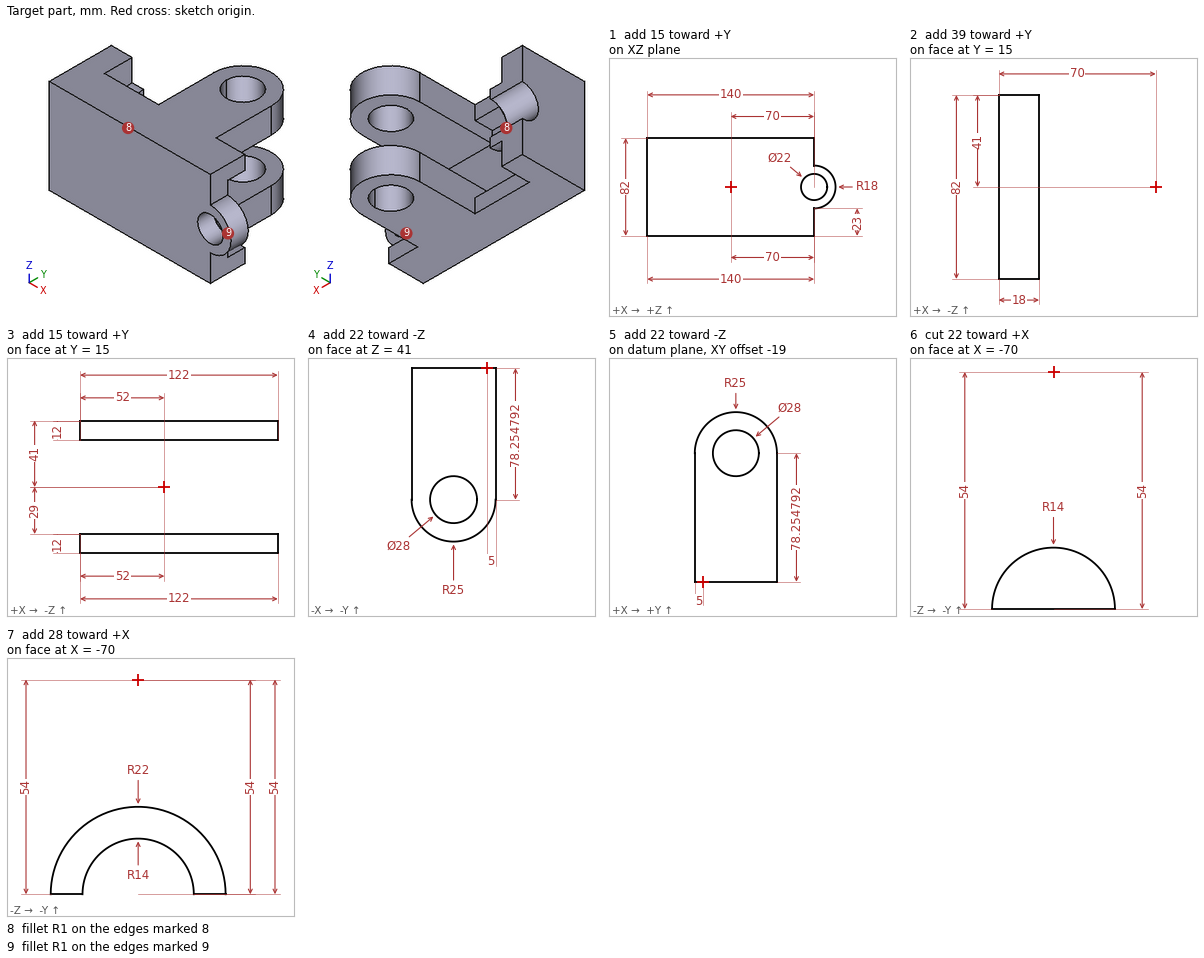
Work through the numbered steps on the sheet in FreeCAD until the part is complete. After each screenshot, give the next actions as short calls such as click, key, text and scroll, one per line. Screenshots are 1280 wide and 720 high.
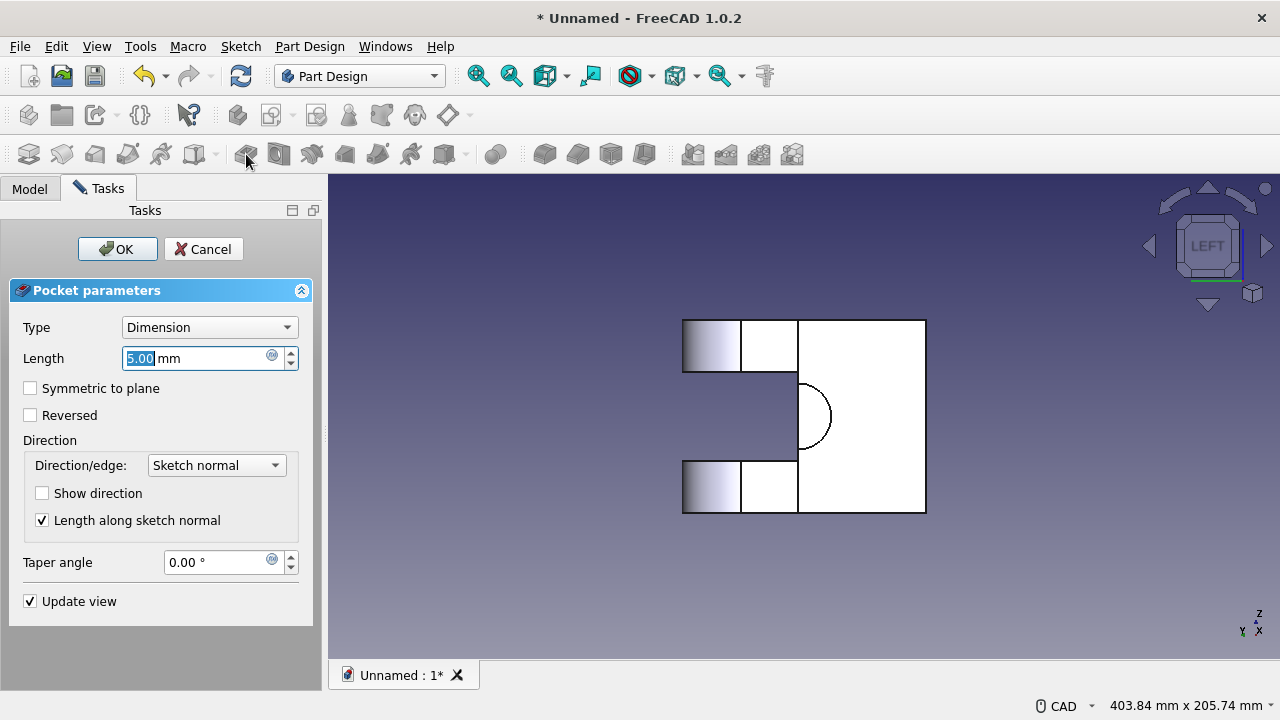
text(22)
key(Tab)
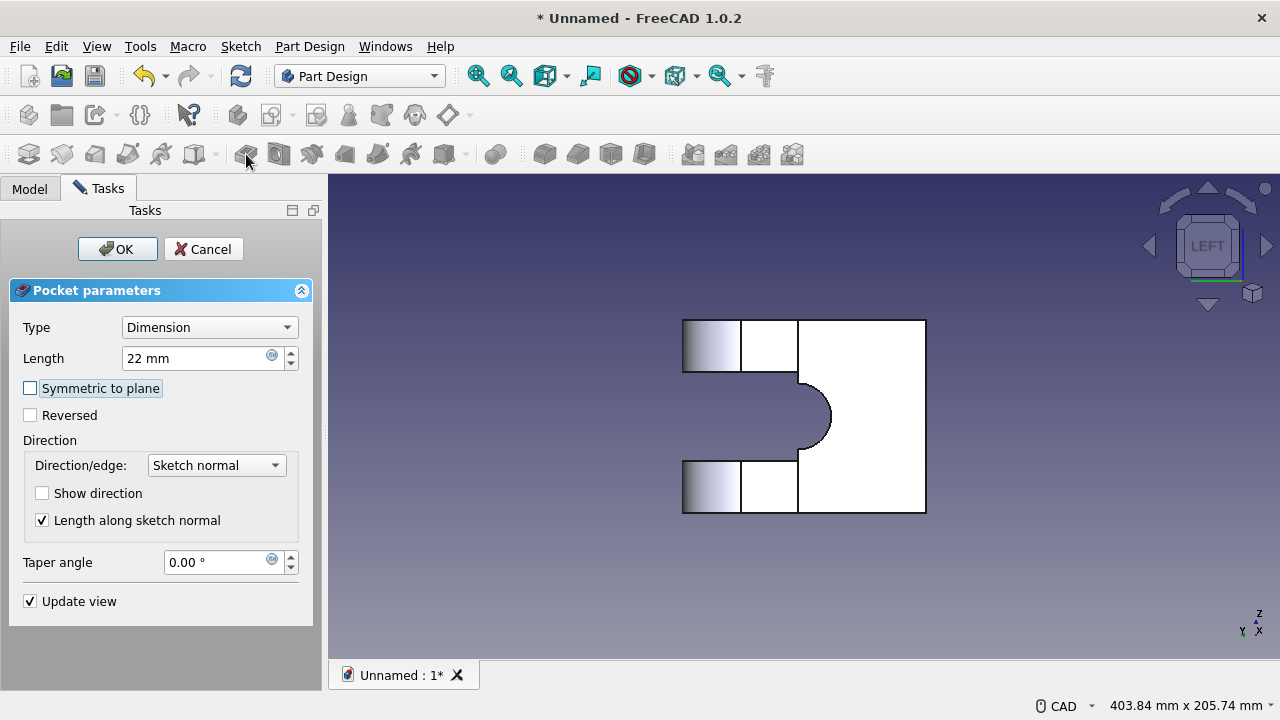
click(118, 249)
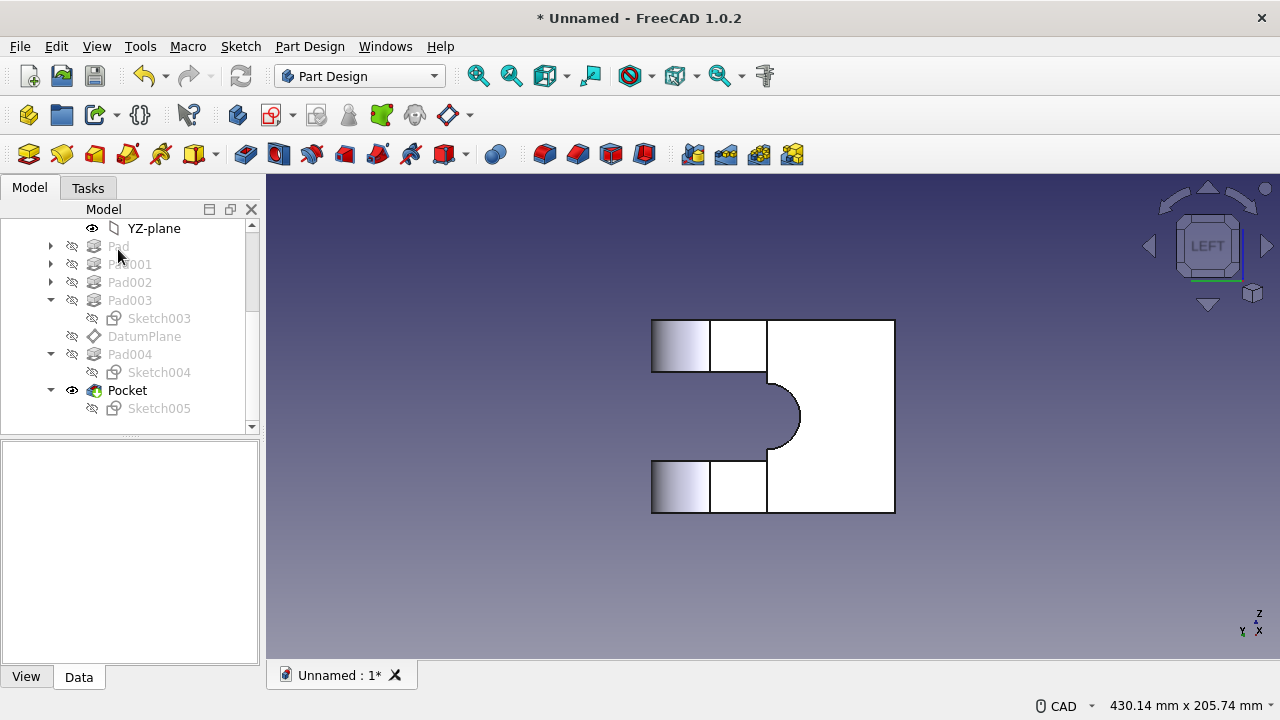
click(479, 76)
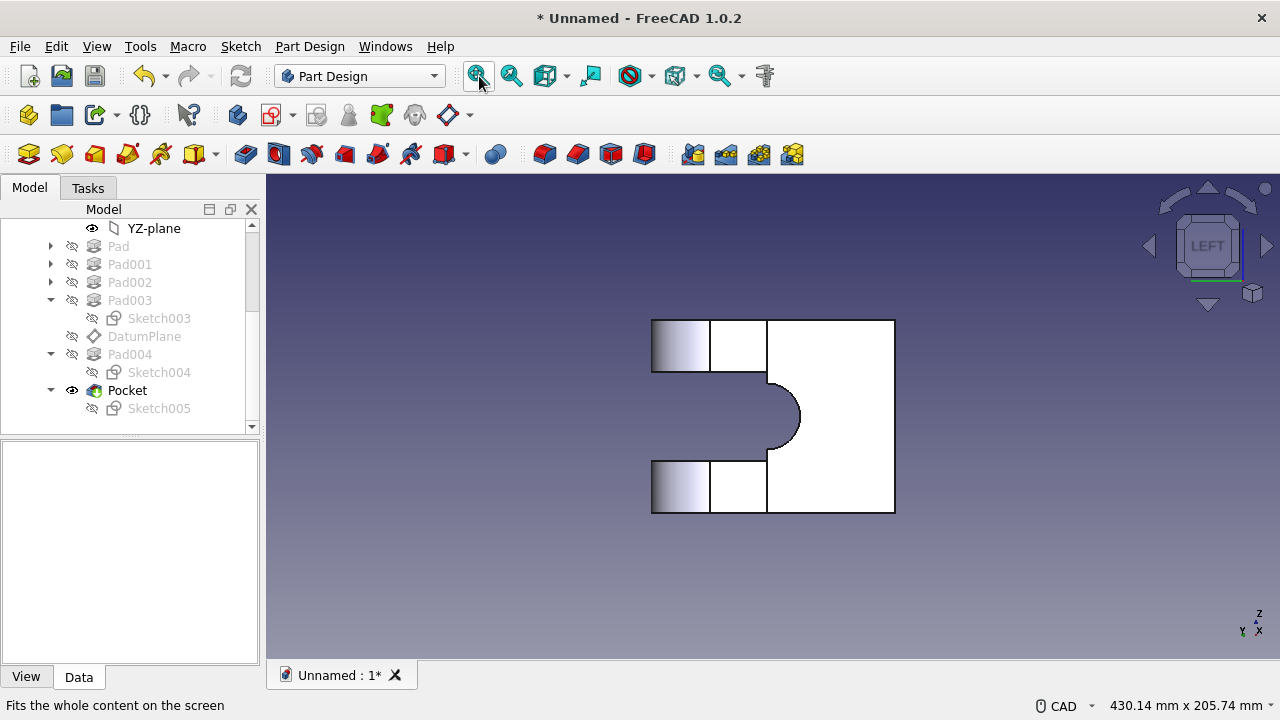
click(849, 443)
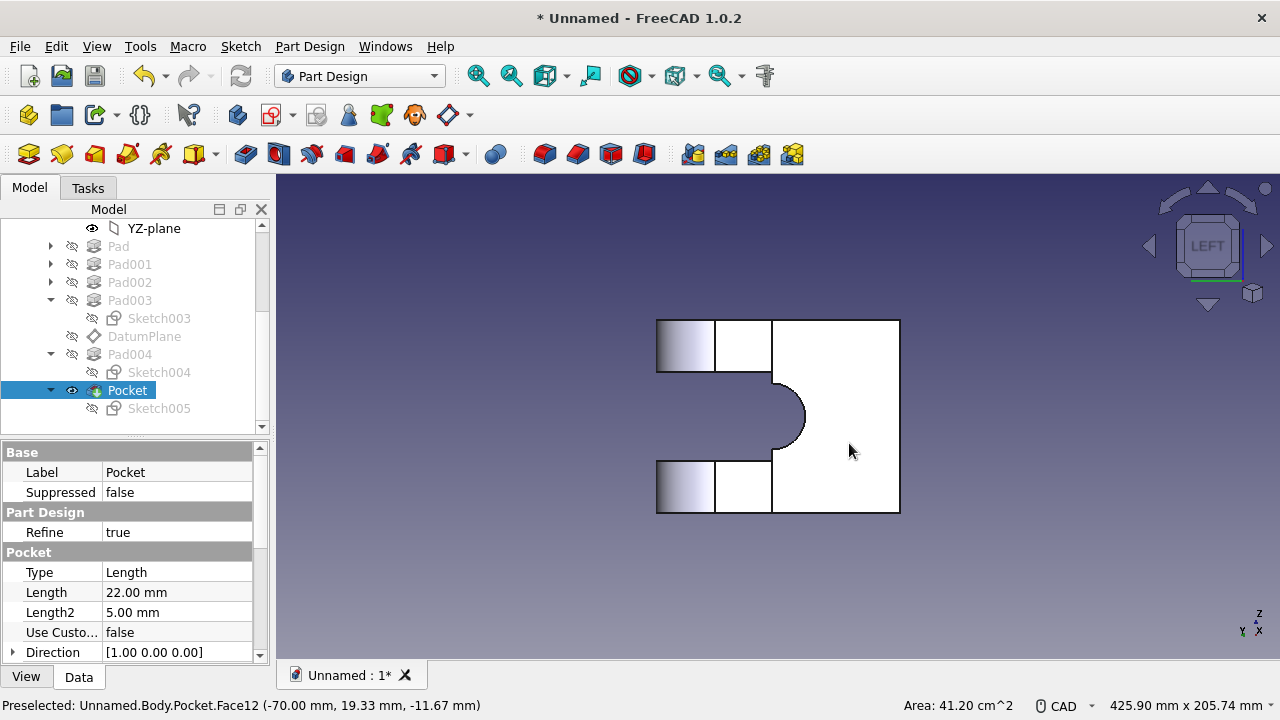
click(270, 116)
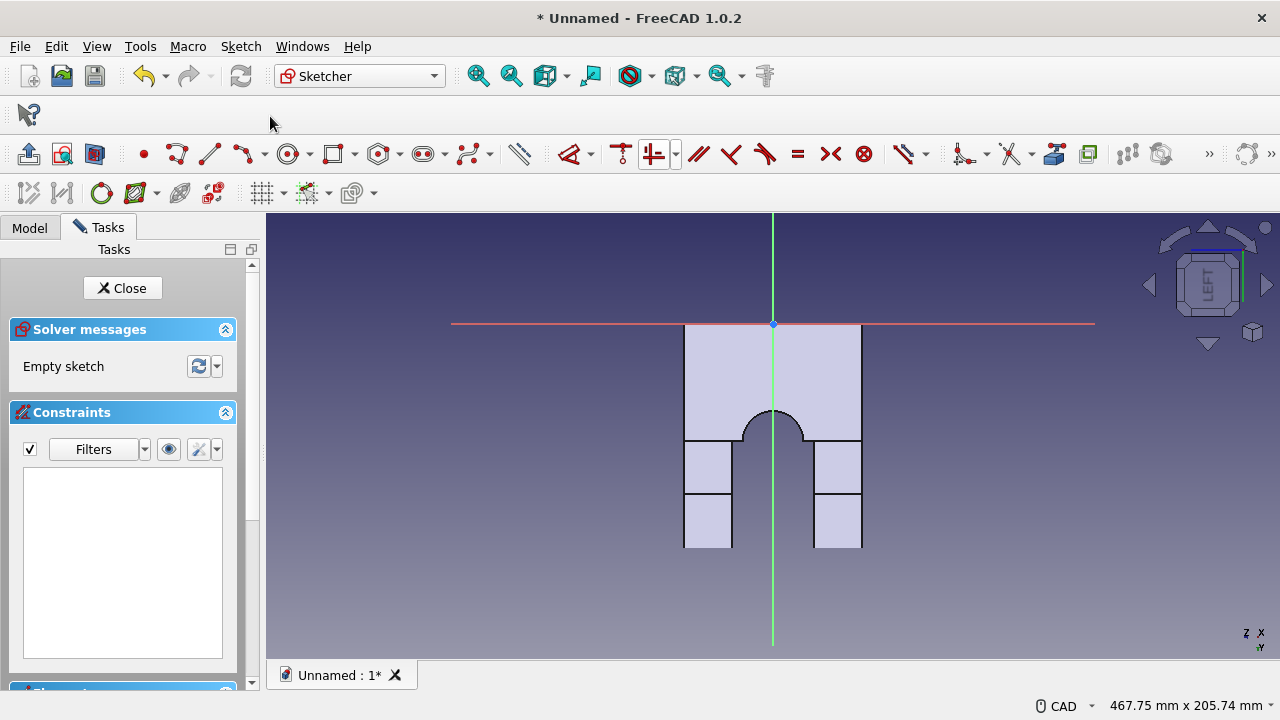
scroll(829, 339, up, 4)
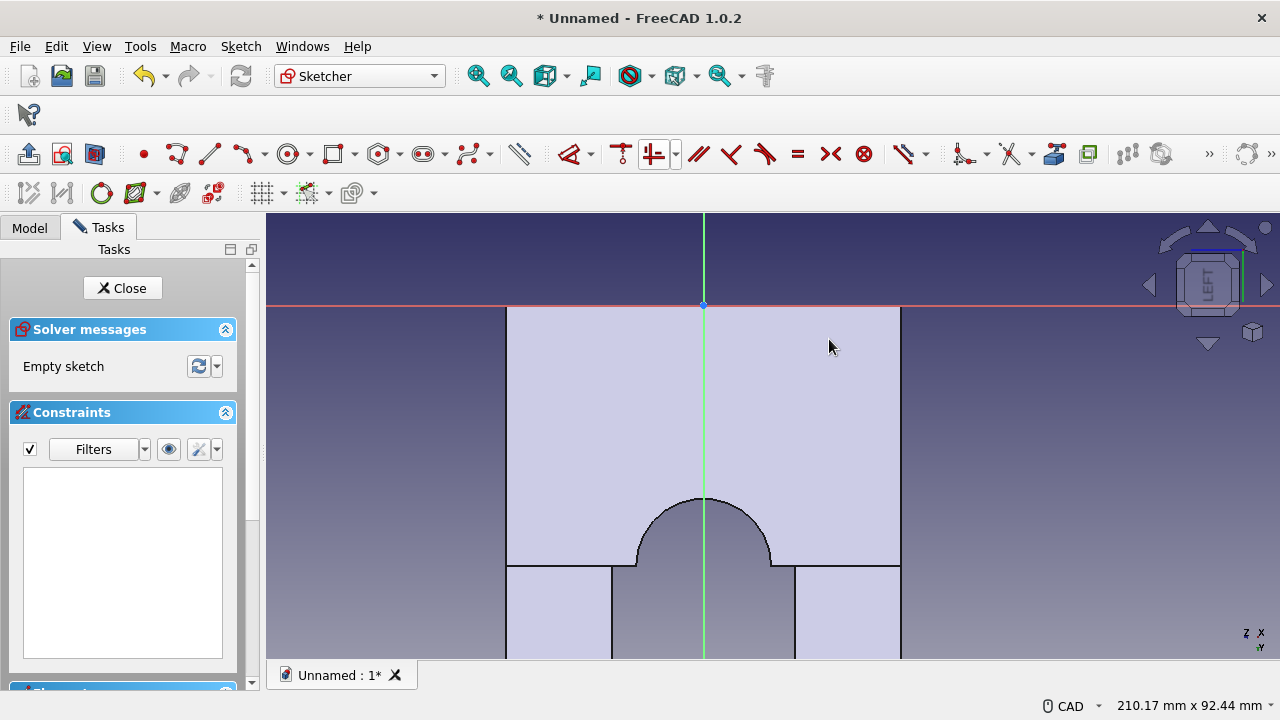
click(210, 154)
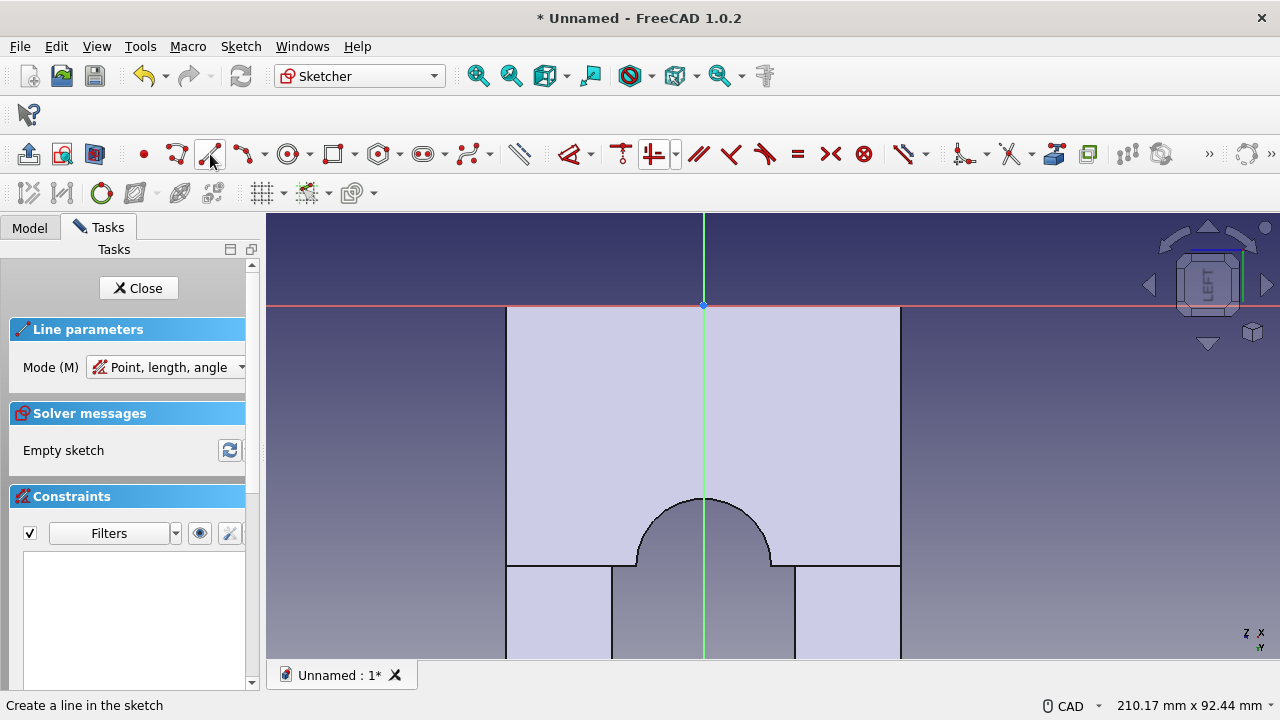
click(771, 566)
click(810, 566)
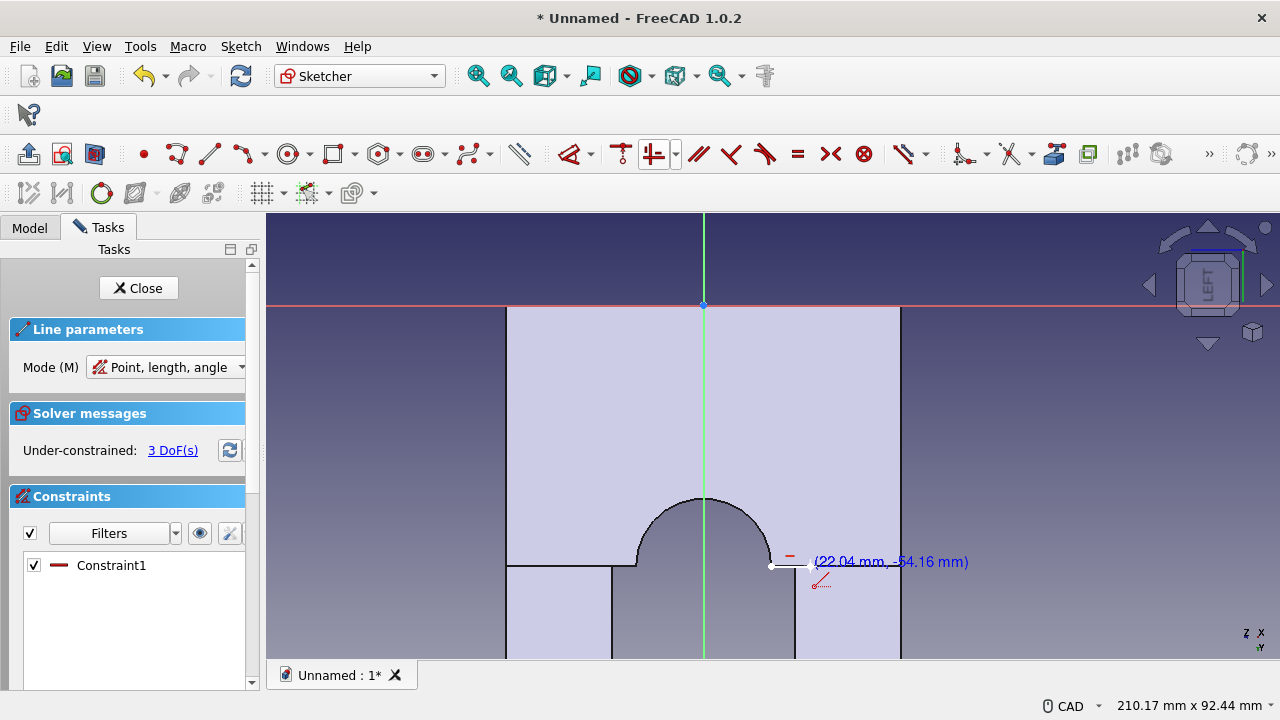
click(598, 566)
click(636, 566)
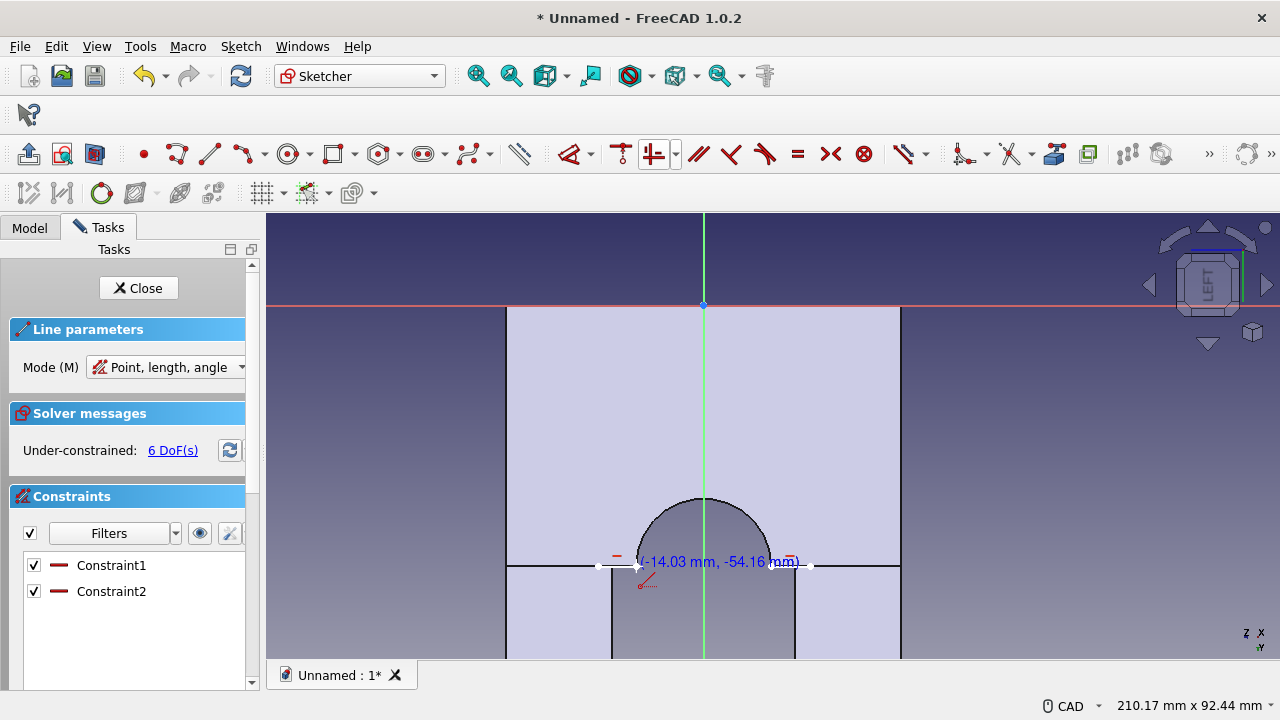
click(242, 154)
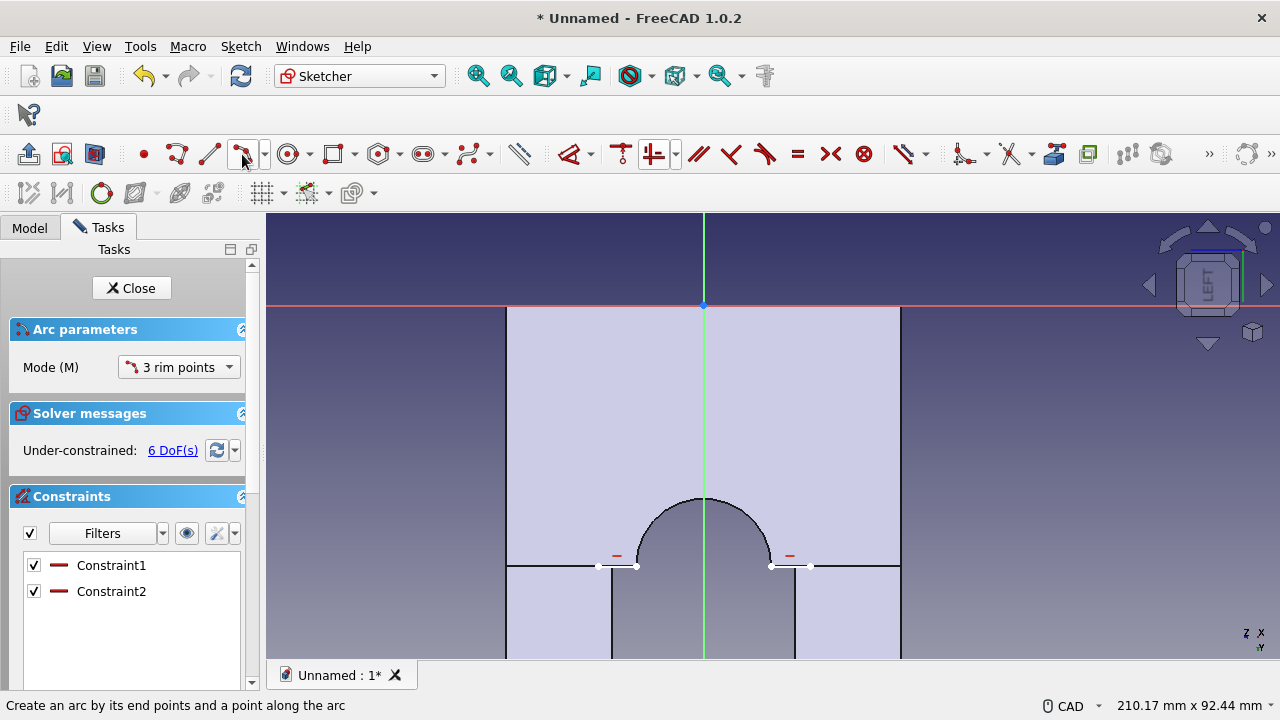
click(810, 567)
click(598, 567)
click(736, 465)